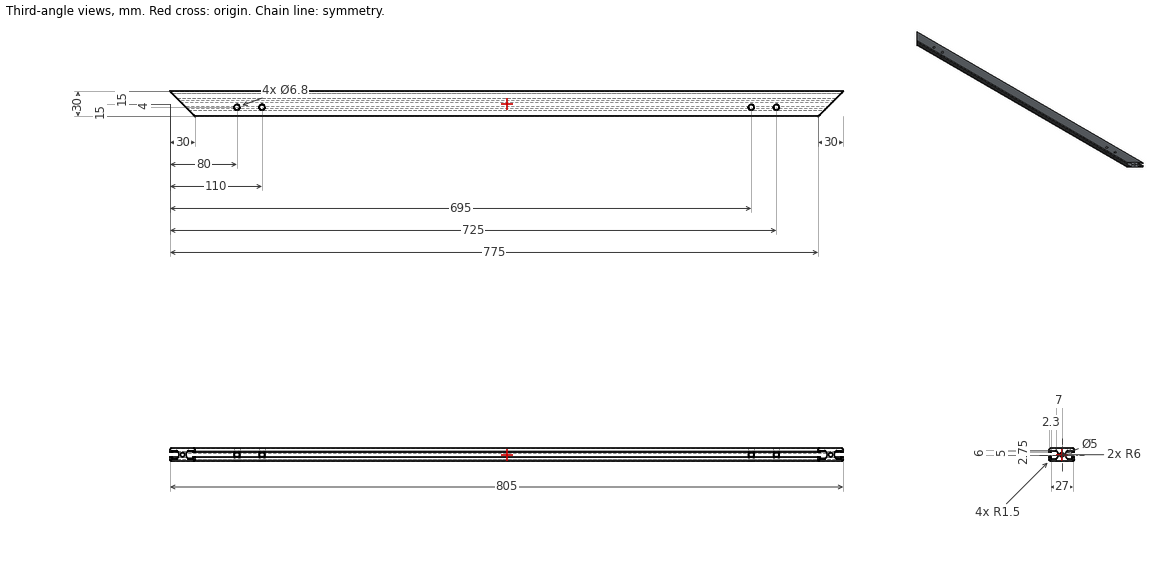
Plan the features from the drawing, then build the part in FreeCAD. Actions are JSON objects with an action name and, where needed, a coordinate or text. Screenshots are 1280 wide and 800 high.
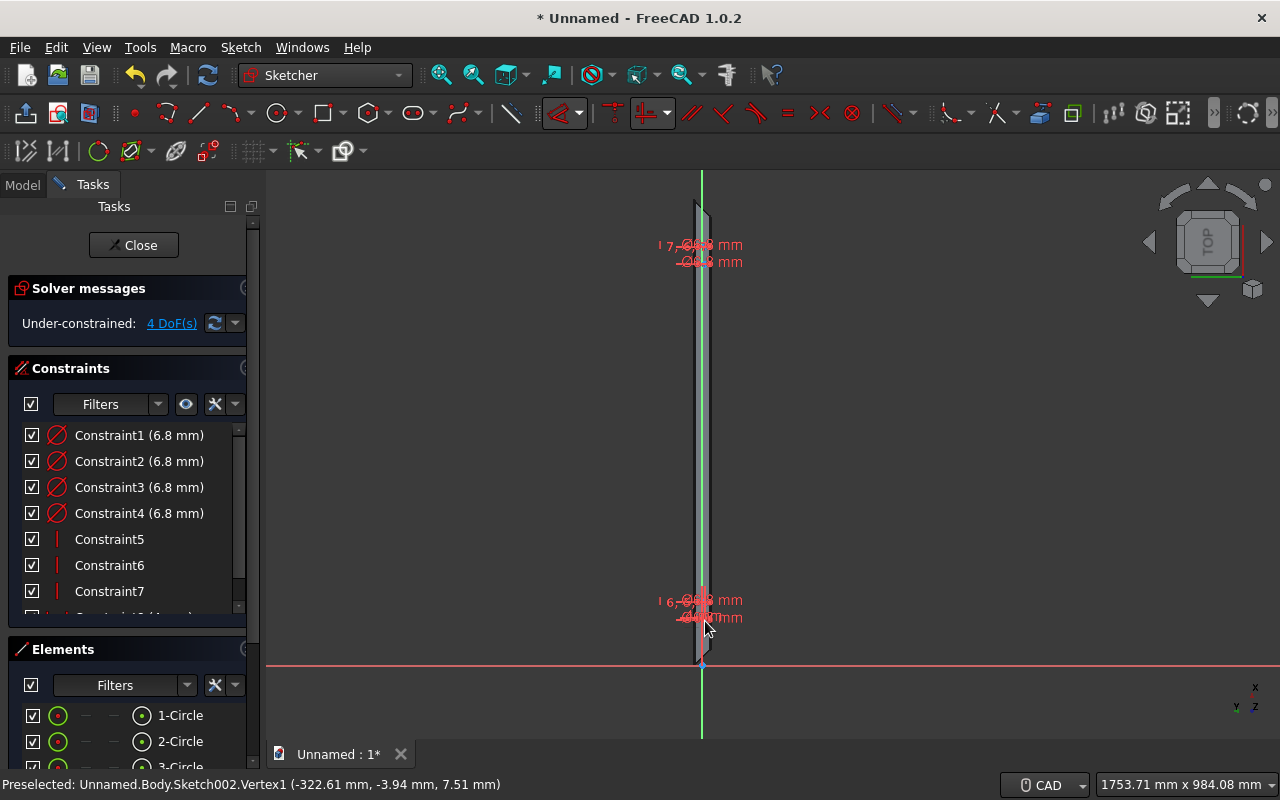
{"action": "left_click", "coordinate": [705, 620]}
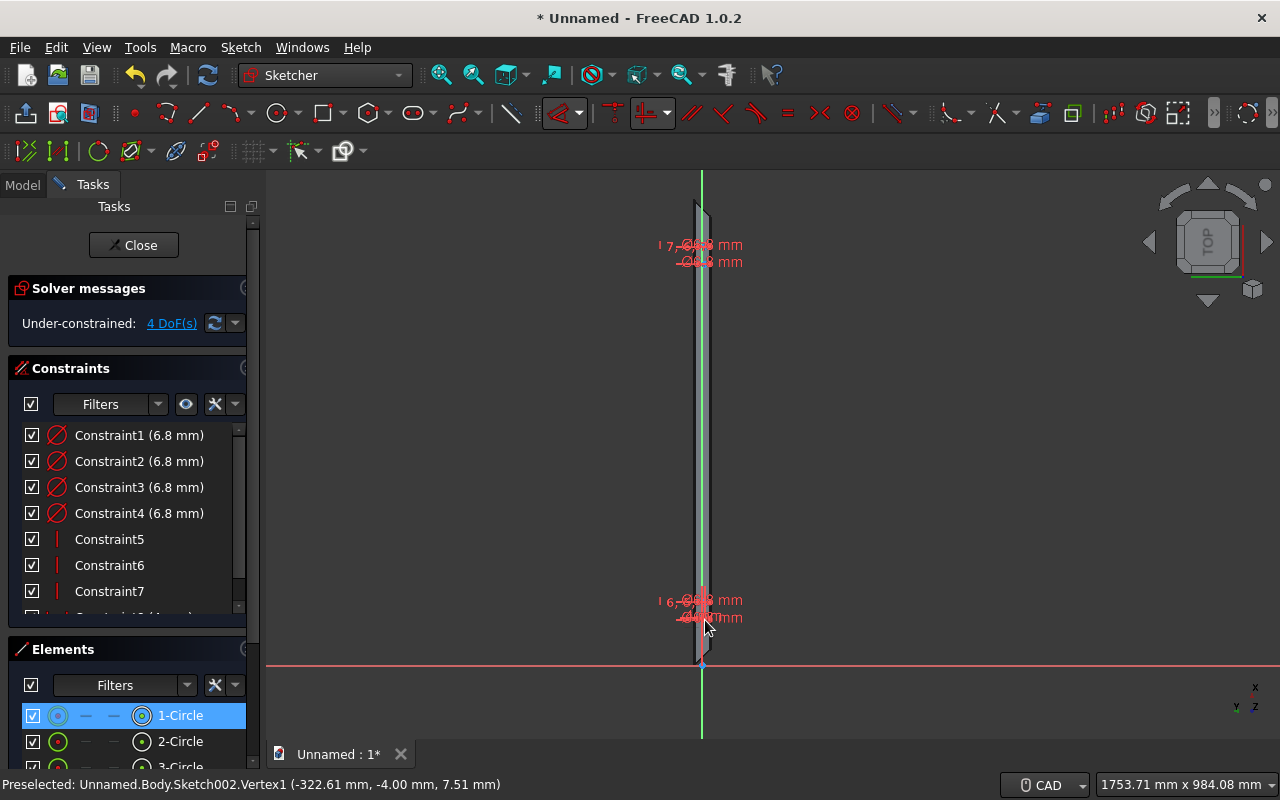
{"action": "left_click", "coordinate": [582, 114]}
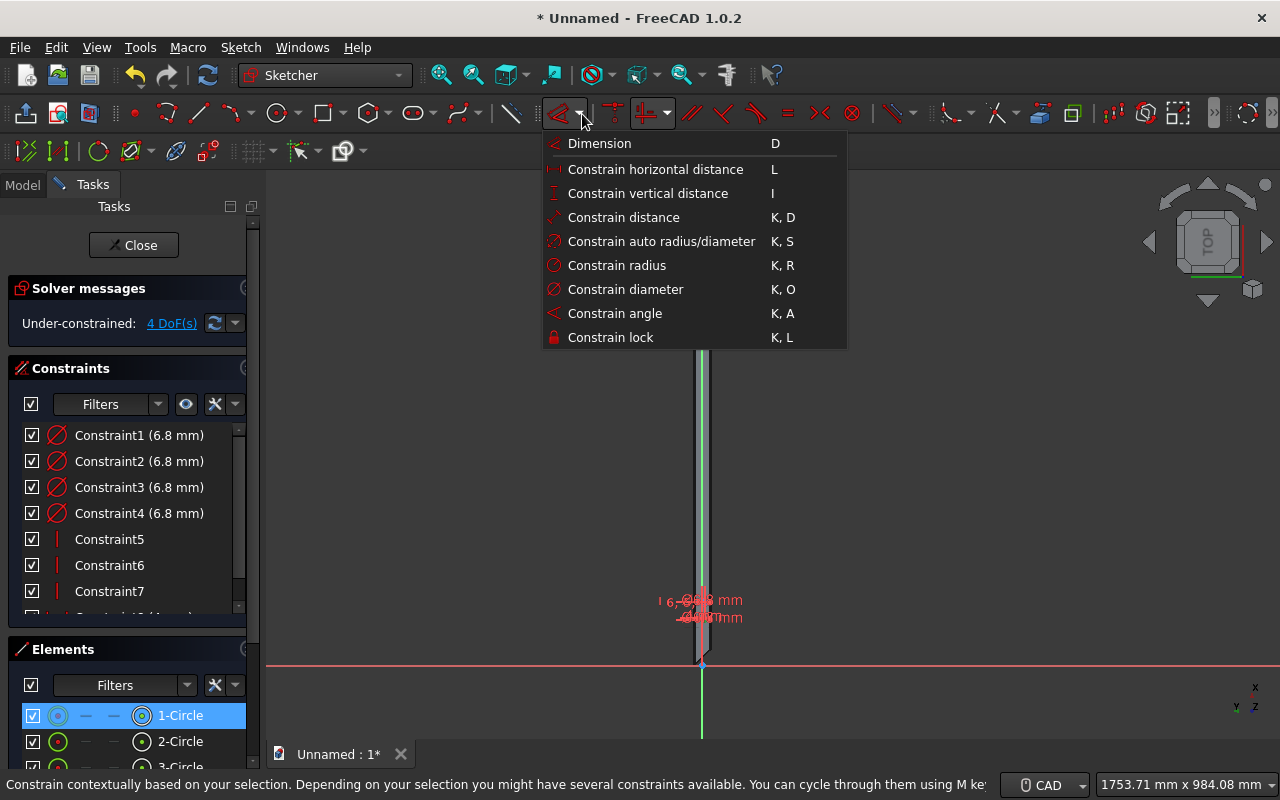
{"action": "left_click", "coordinate": [695, 193]}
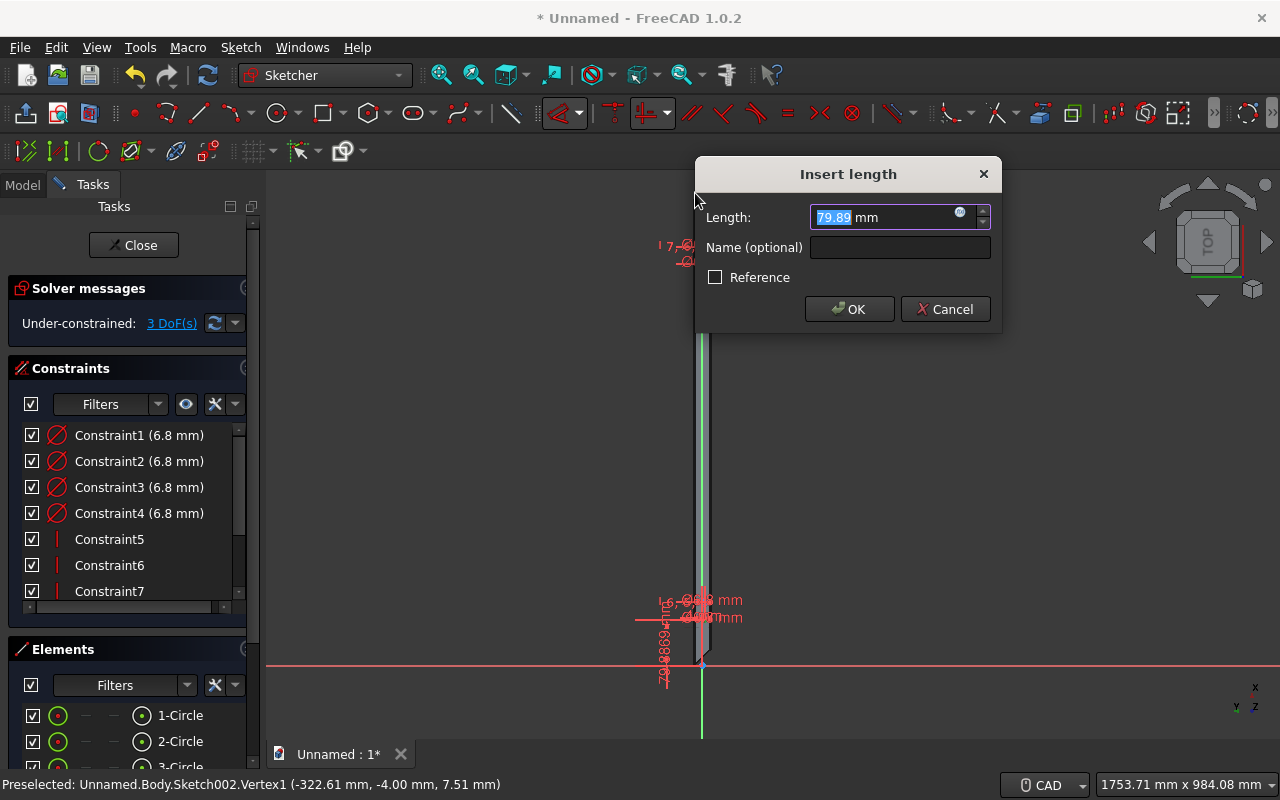
{"action": "type", "text": "80"}
{"action": "key", "text": "Return"}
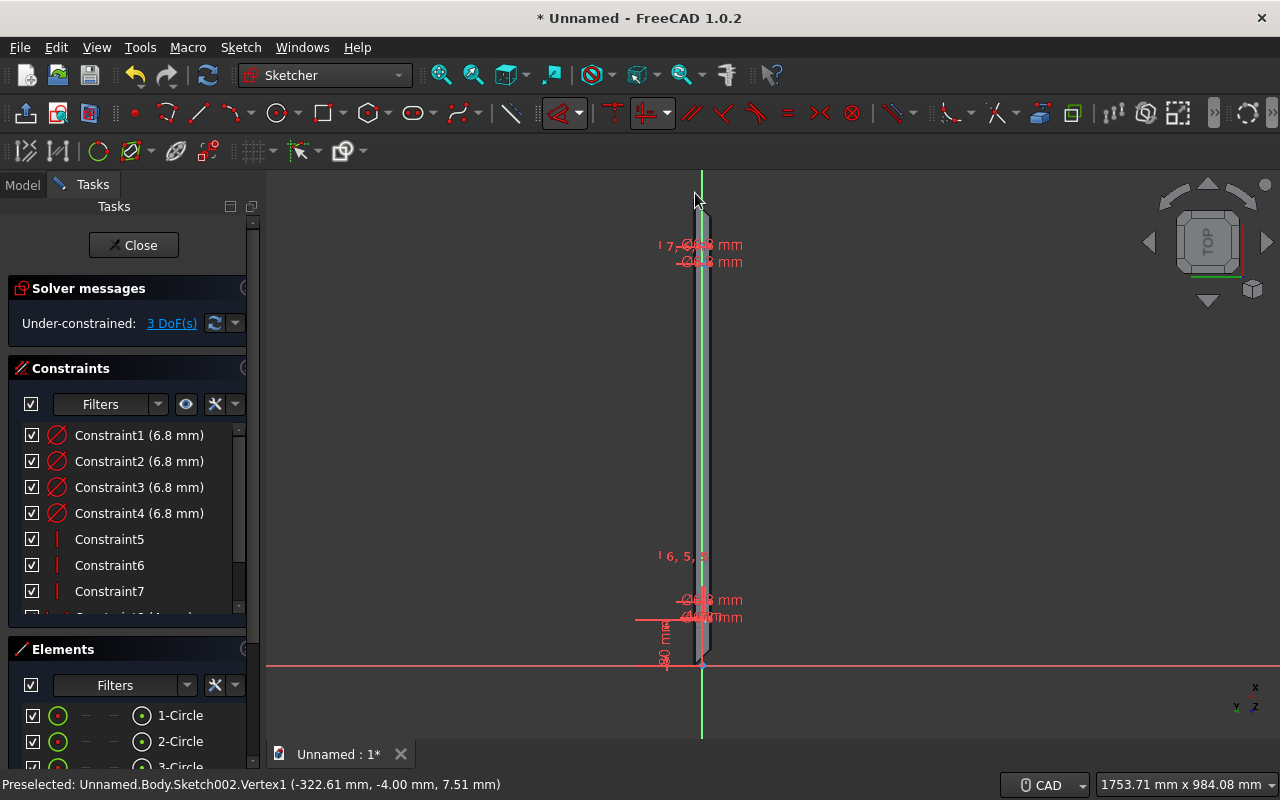
{"action": "left_click", "coordinate": [705, 602]}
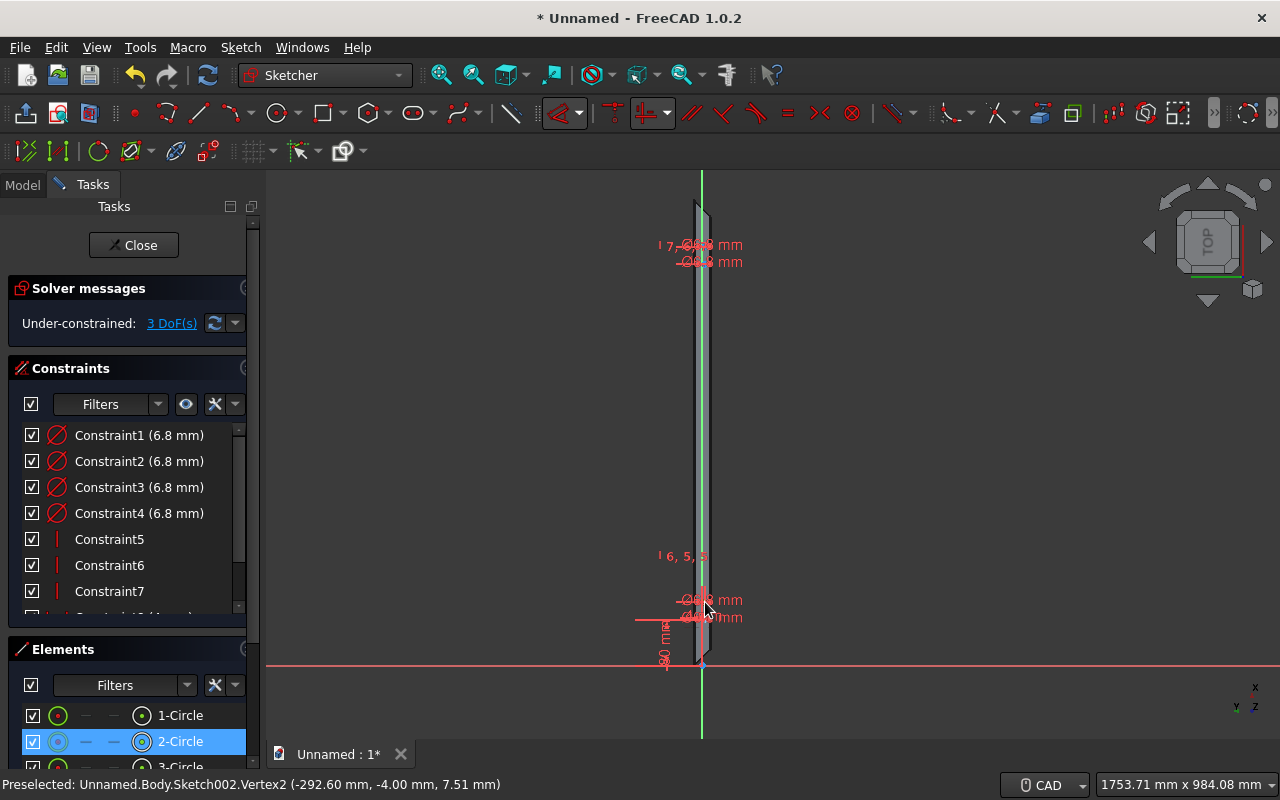
{"action": "left_click", "coordinate": [582, 114]}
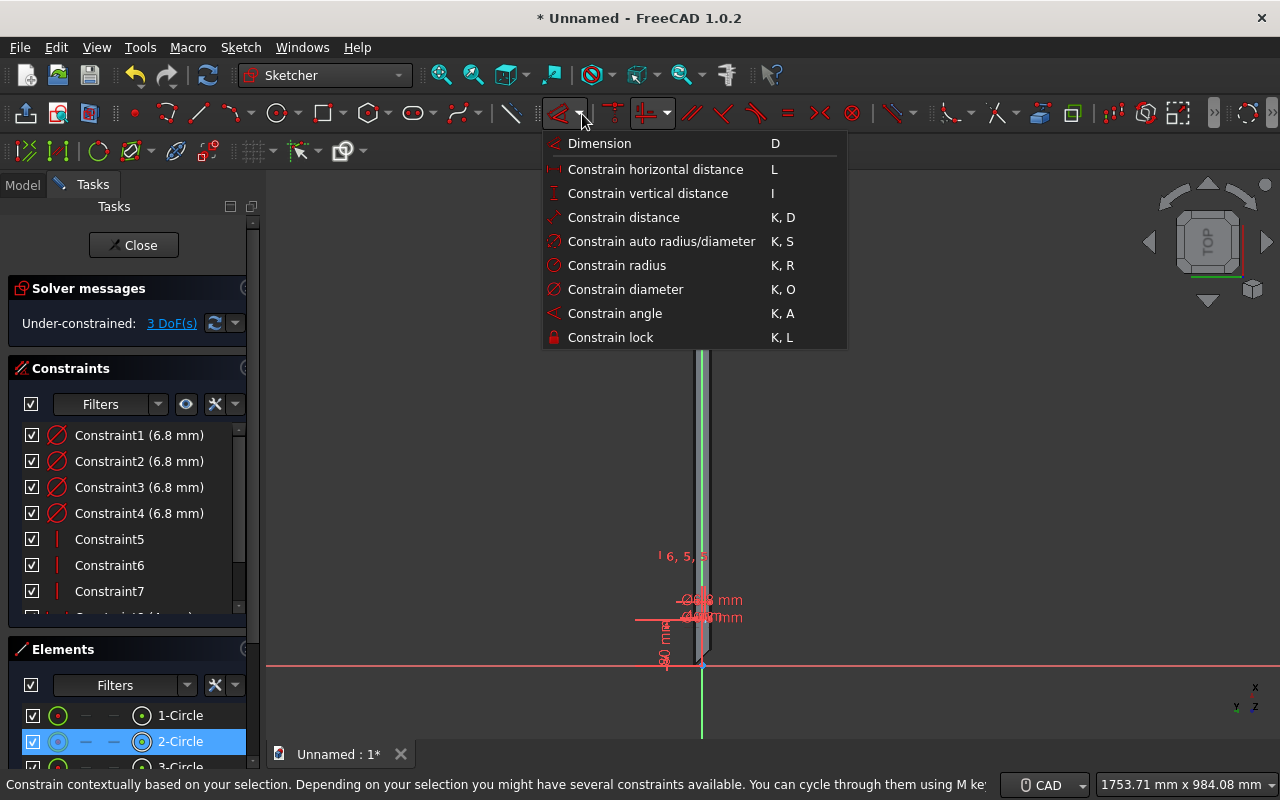
{"action": "left_click", "coordinate": [695, 193]}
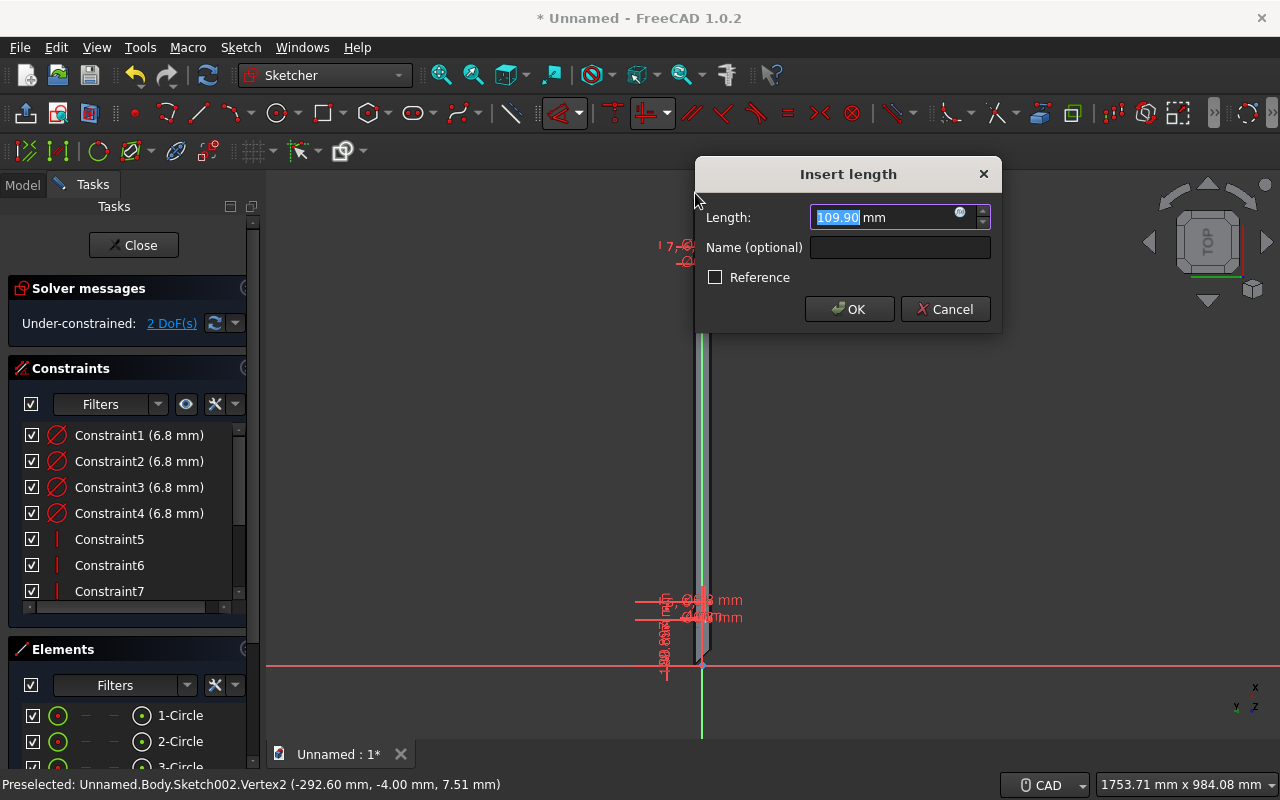
{"action": "type", "text": "110"}
{"action": "key", "text": "Return"}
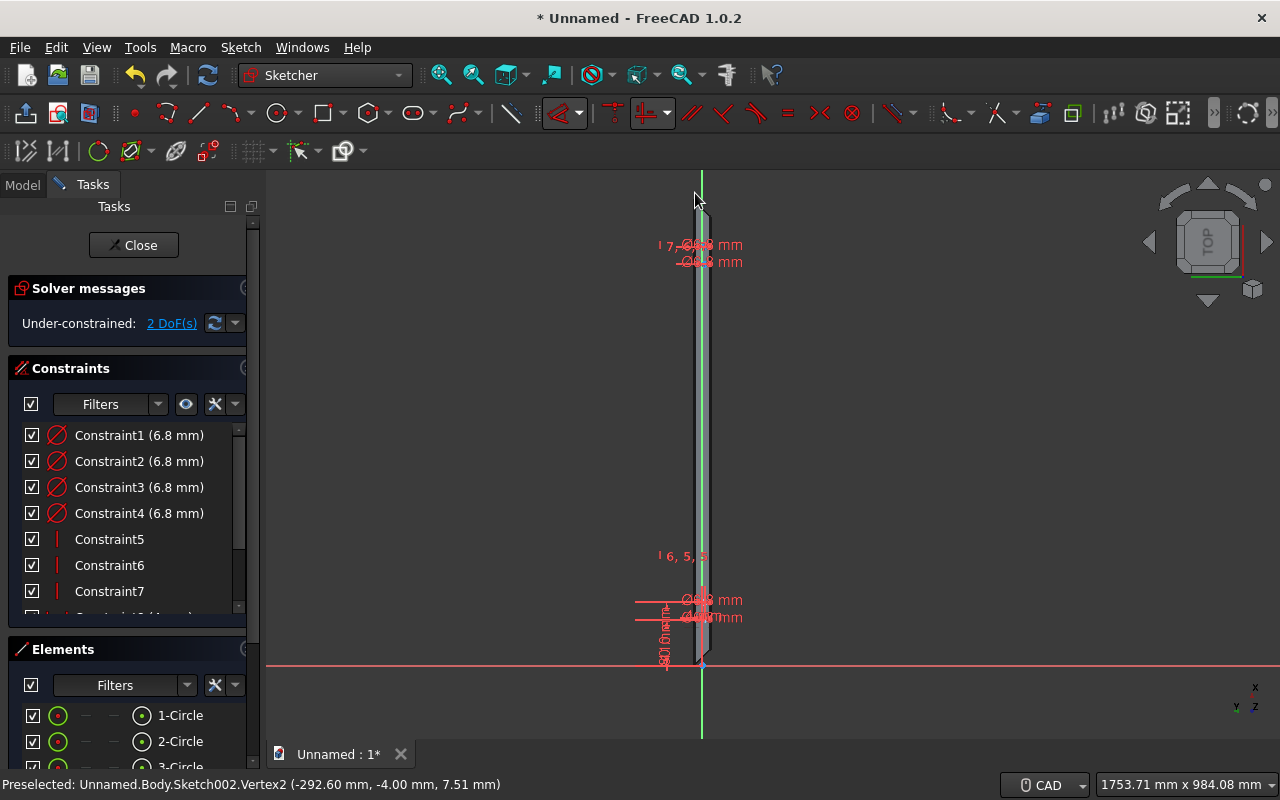
{"action": "left_click", "coordinate": [705, 264]}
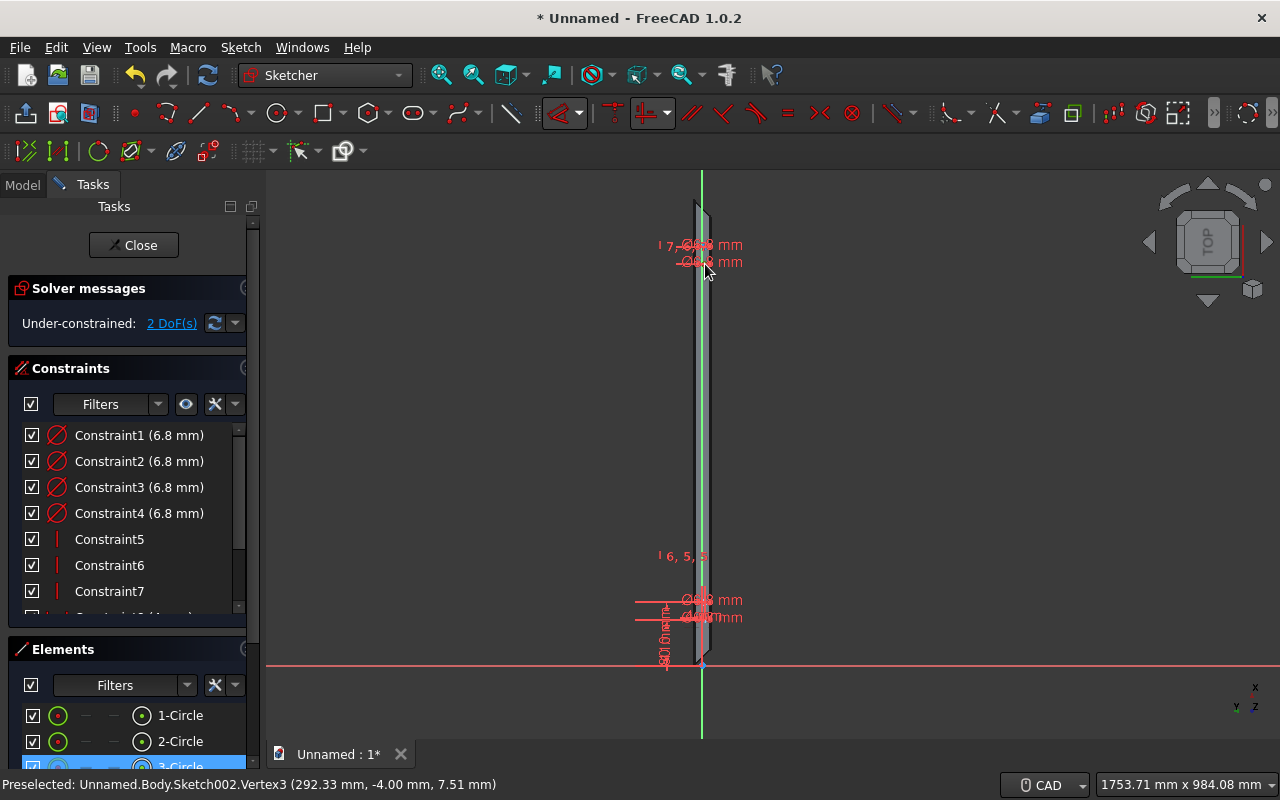
{"action": "key", "text": "i"}